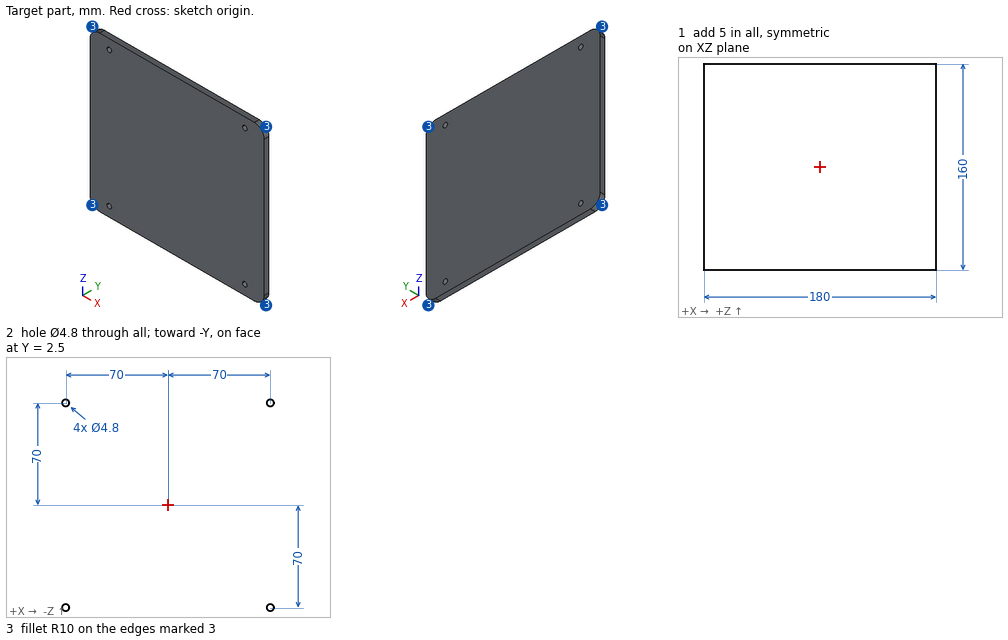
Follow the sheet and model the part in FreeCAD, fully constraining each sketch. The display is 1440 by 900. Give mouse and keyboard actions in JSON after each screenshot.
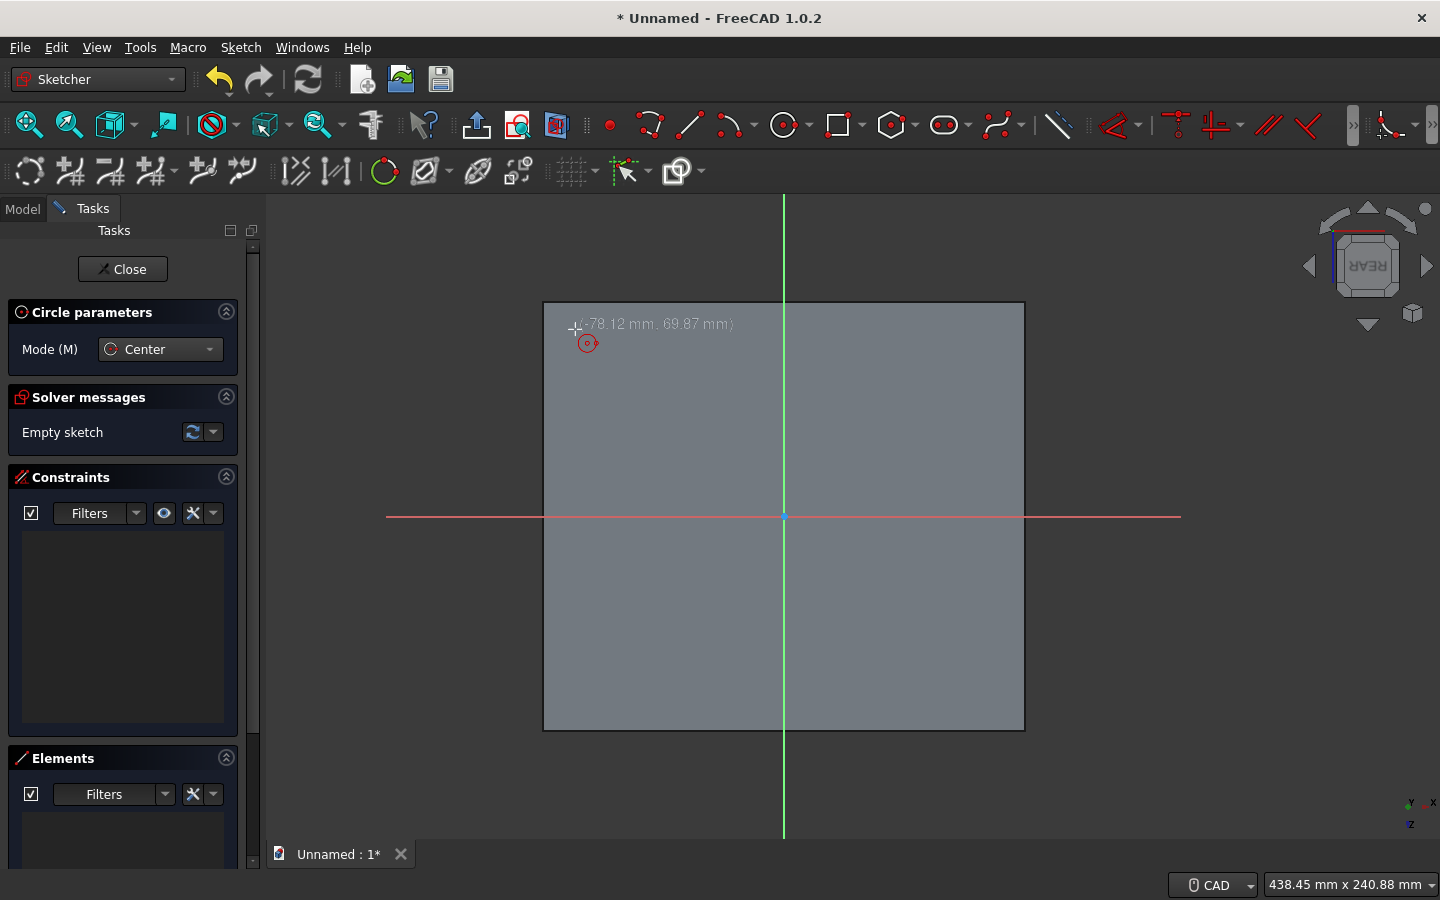
{"action": "left_click", "coordinate": [597, 329]}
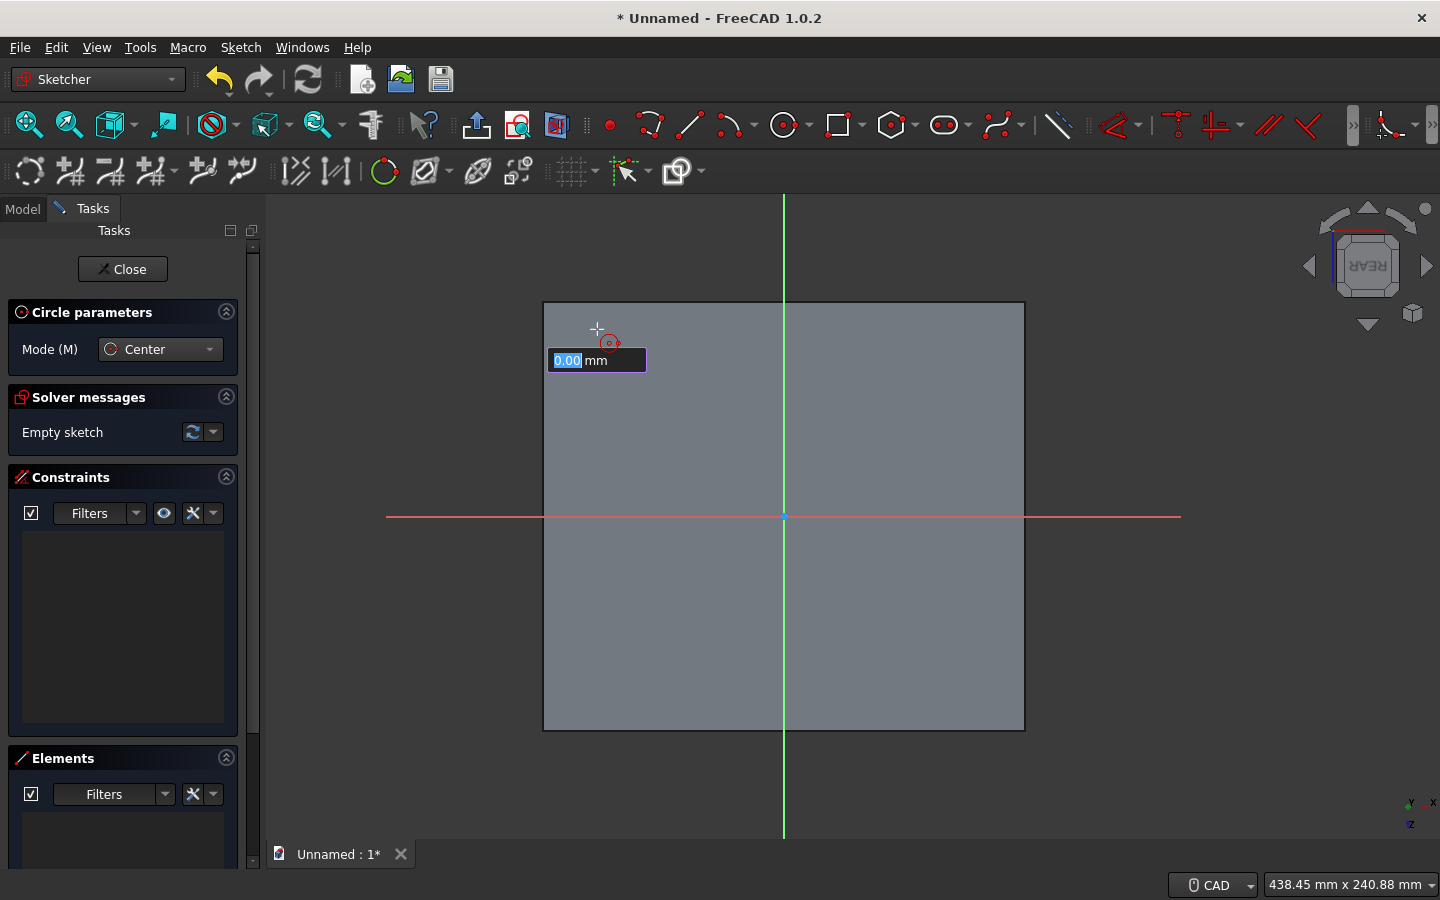
{"action": "scroll", "coordinate": [601, 325], "scroll_direction": "up", "scroll_amount": 5}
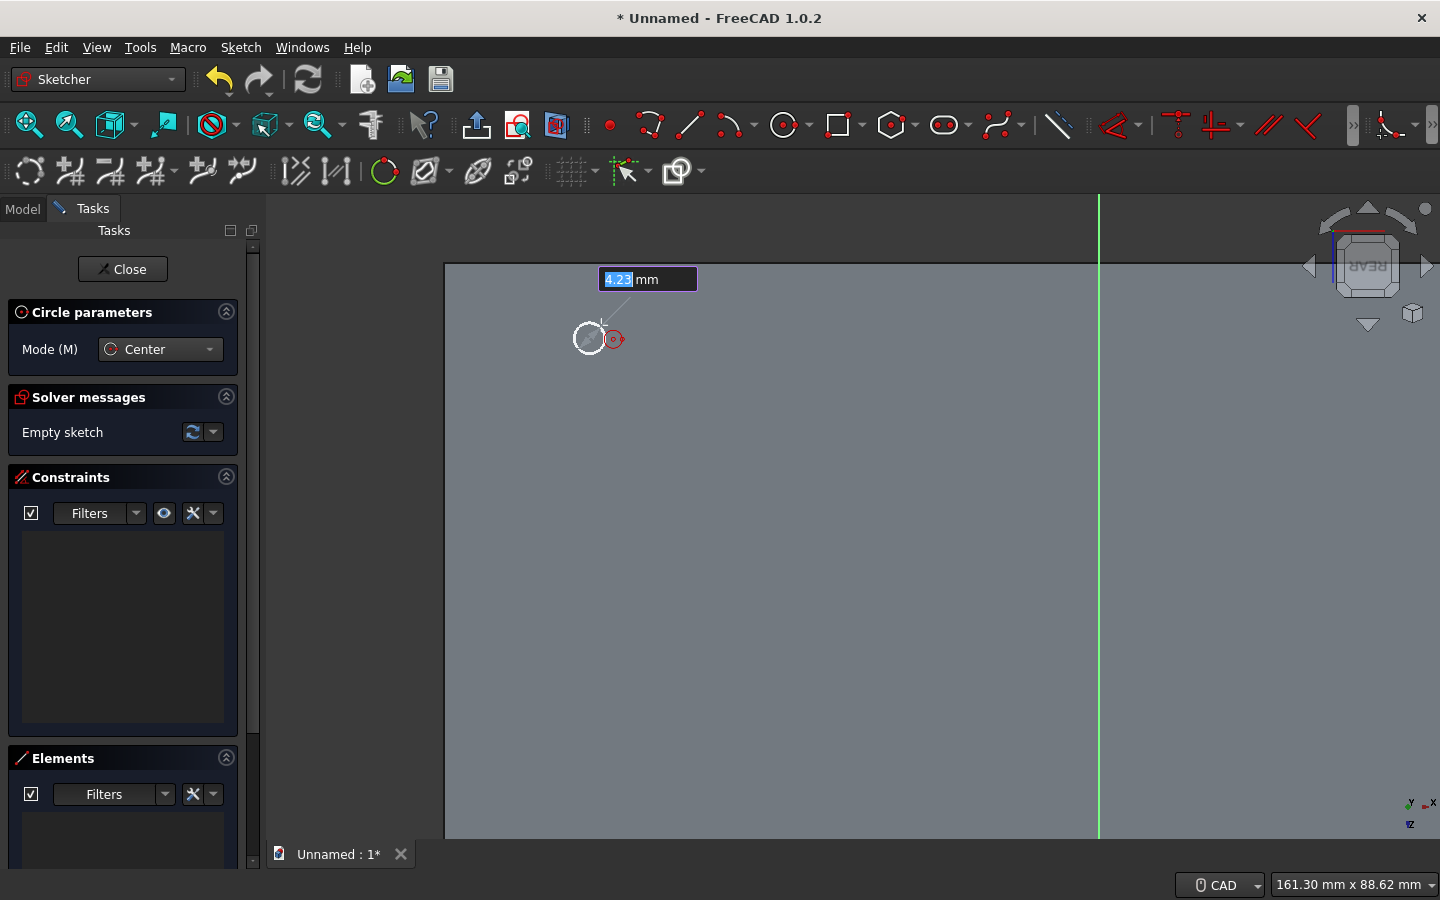
{"action": "left_click", "coordinate": [602, 323]}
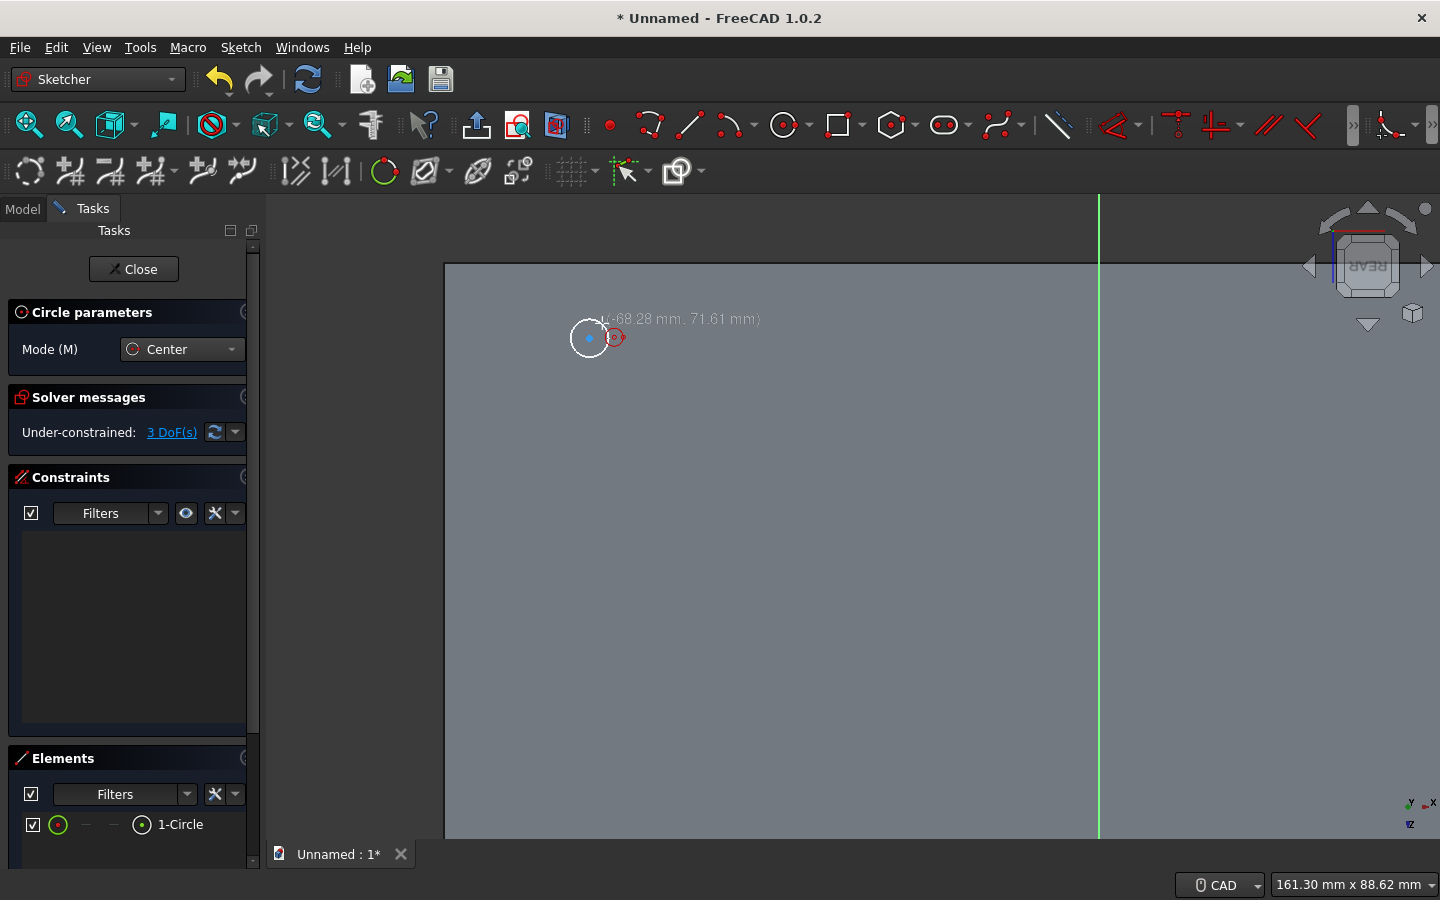
{"action": "scroll", "coordinate": [601, 325], "scroll_direction": "down", "scroll_amount": 5}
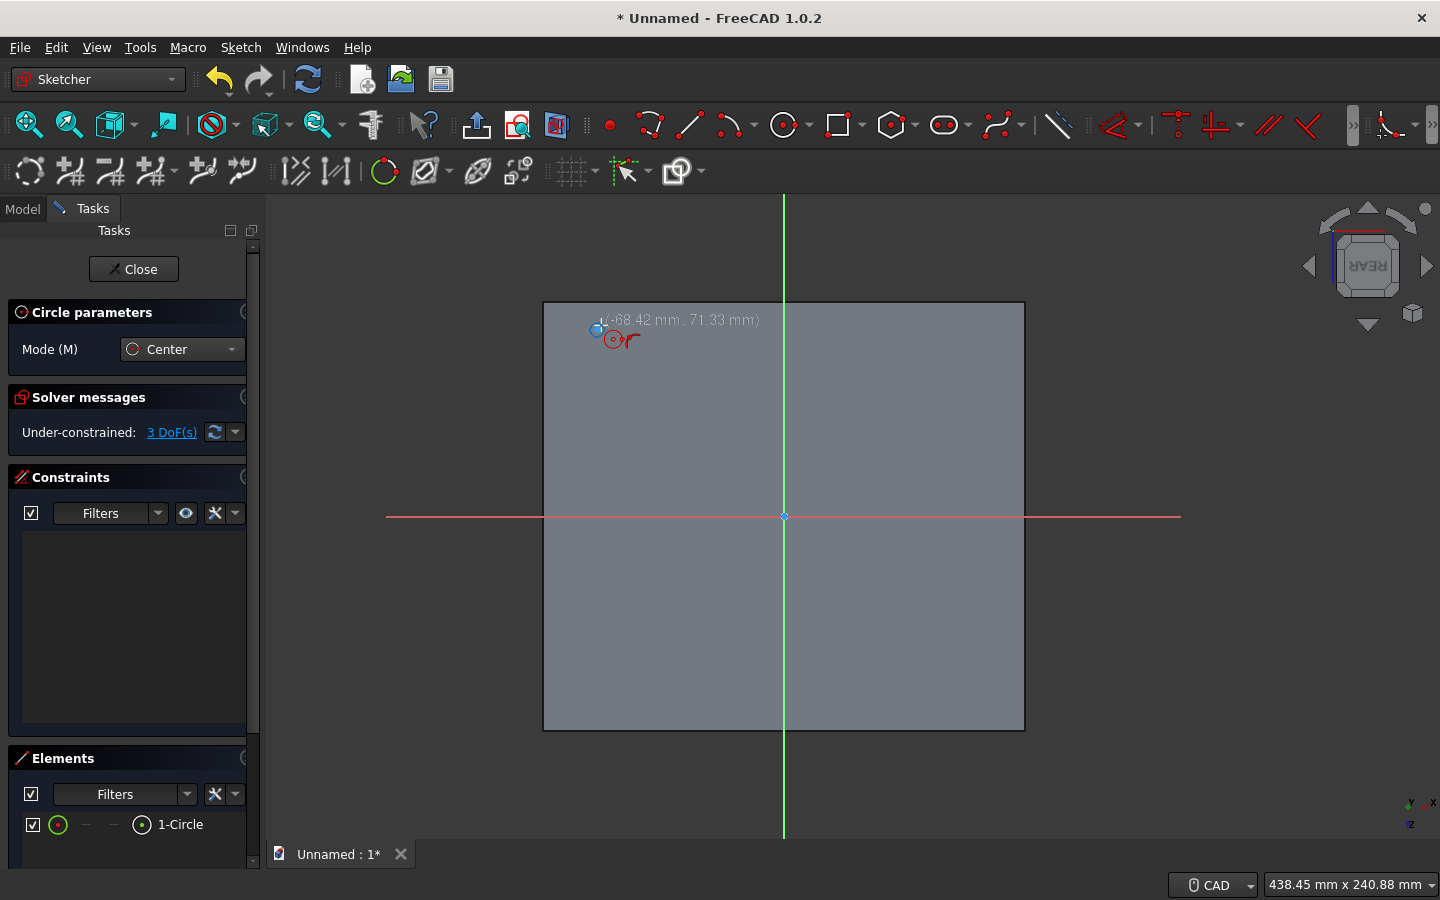
{"action": "scroll", "coordinate": [972, 329], "scroll_direction": "up", "scroll_amount": 7}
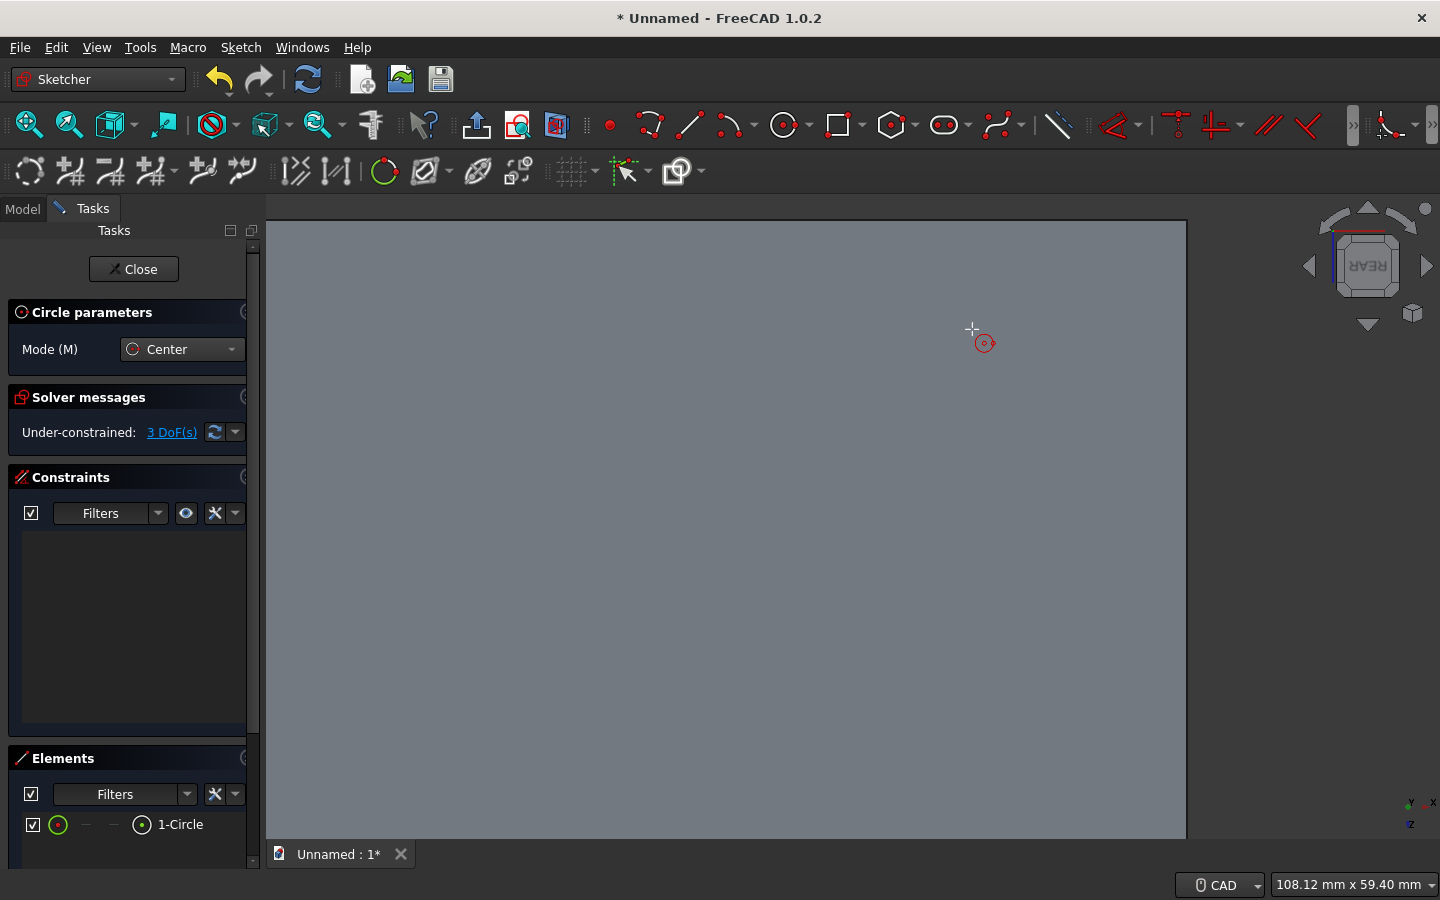
{"action": "scroll", "coordinate": [973, 329], "scroll_direction": "down", "scroll_amount": 7}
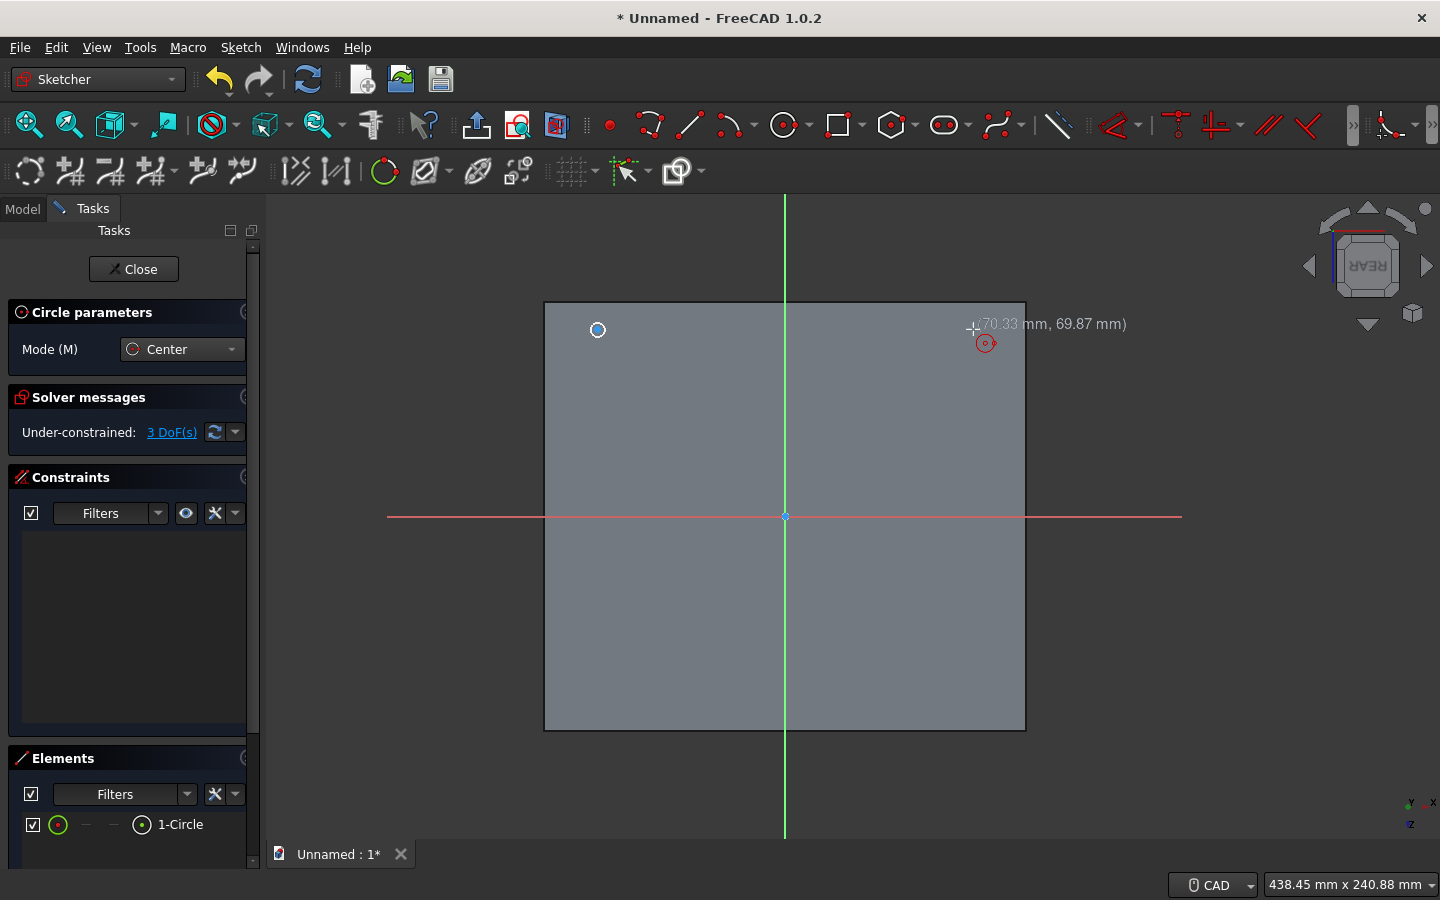
{"action": "left_click", "coordinate": [973, 329]}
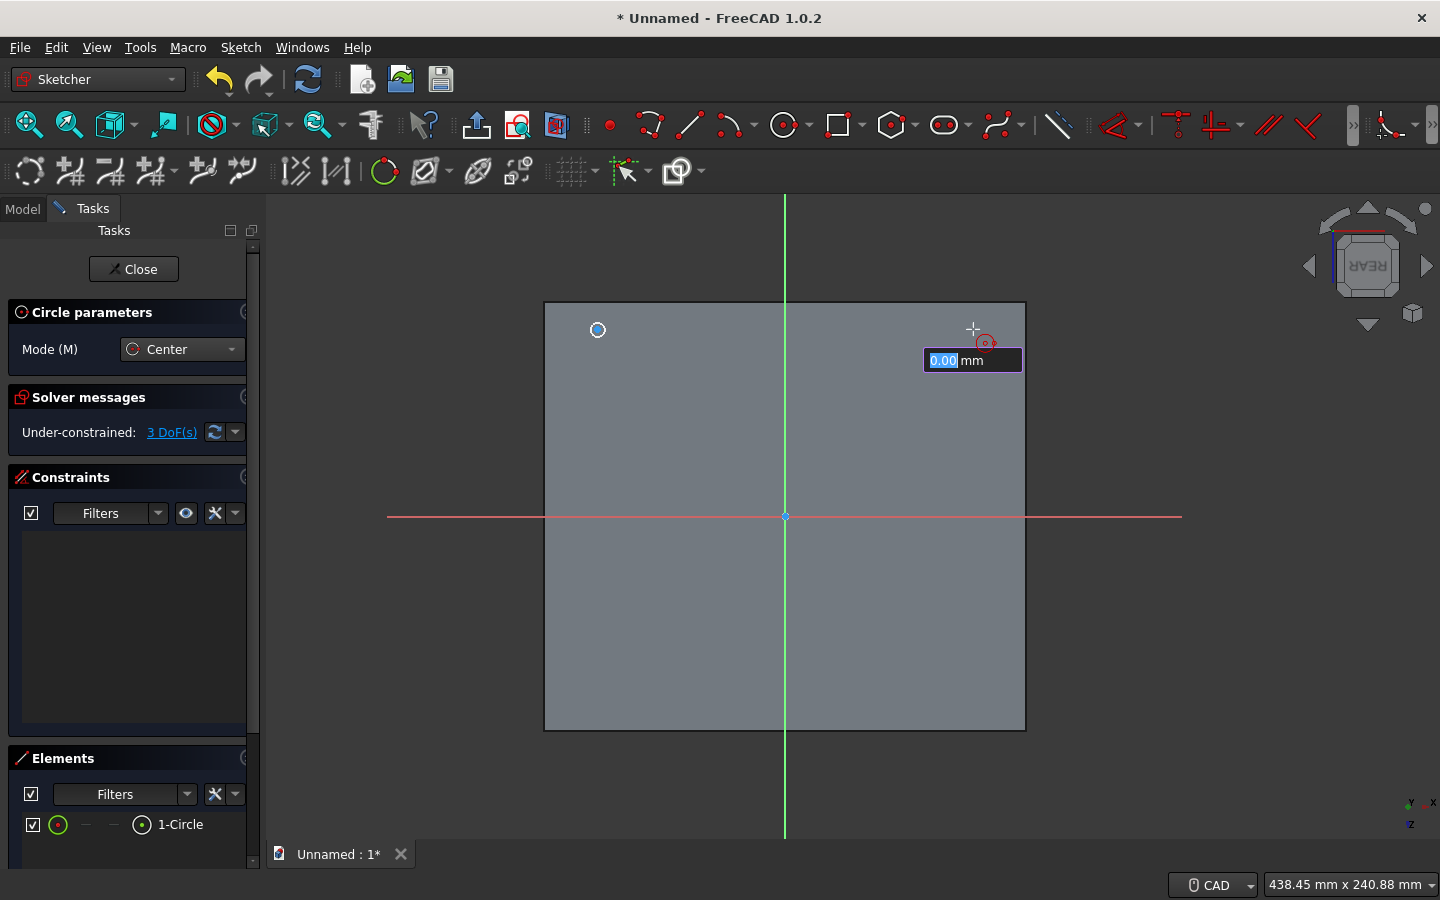
{"action": "scroll", "coordinate": [977, 325], "scroll_direction": "up", "scroll_amount": 5}